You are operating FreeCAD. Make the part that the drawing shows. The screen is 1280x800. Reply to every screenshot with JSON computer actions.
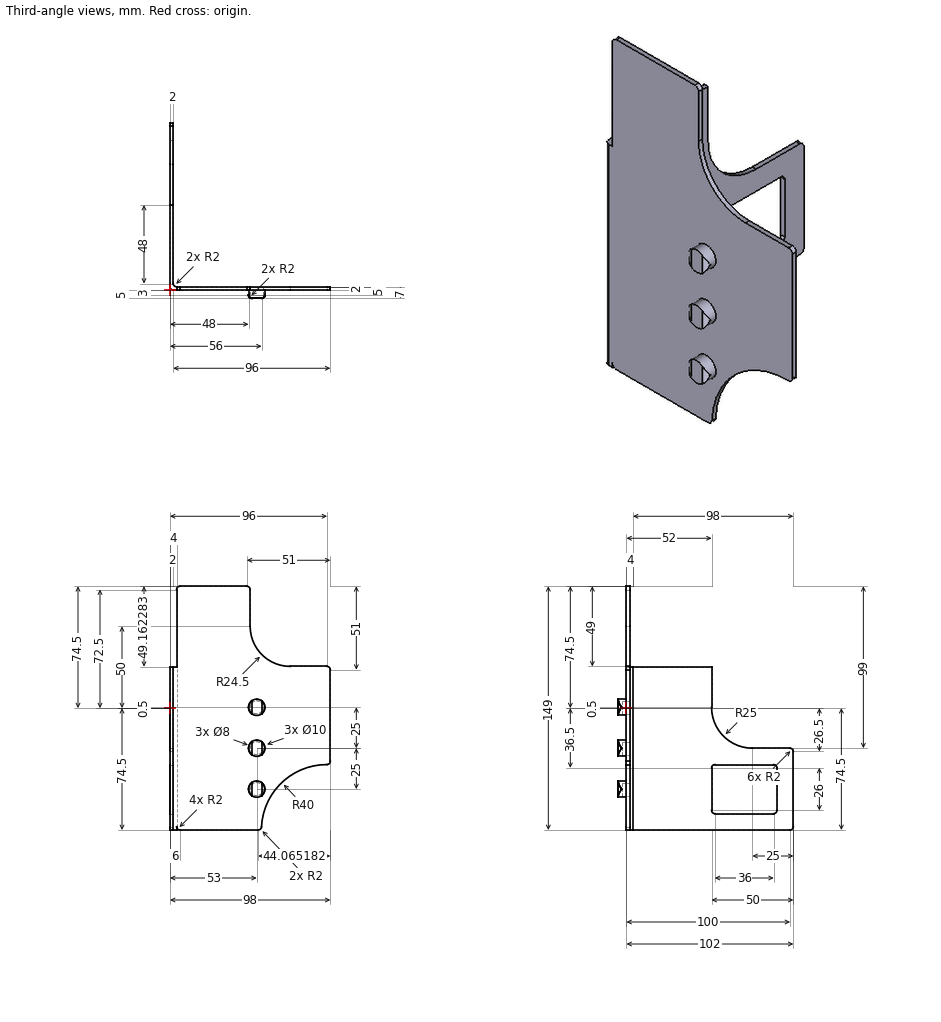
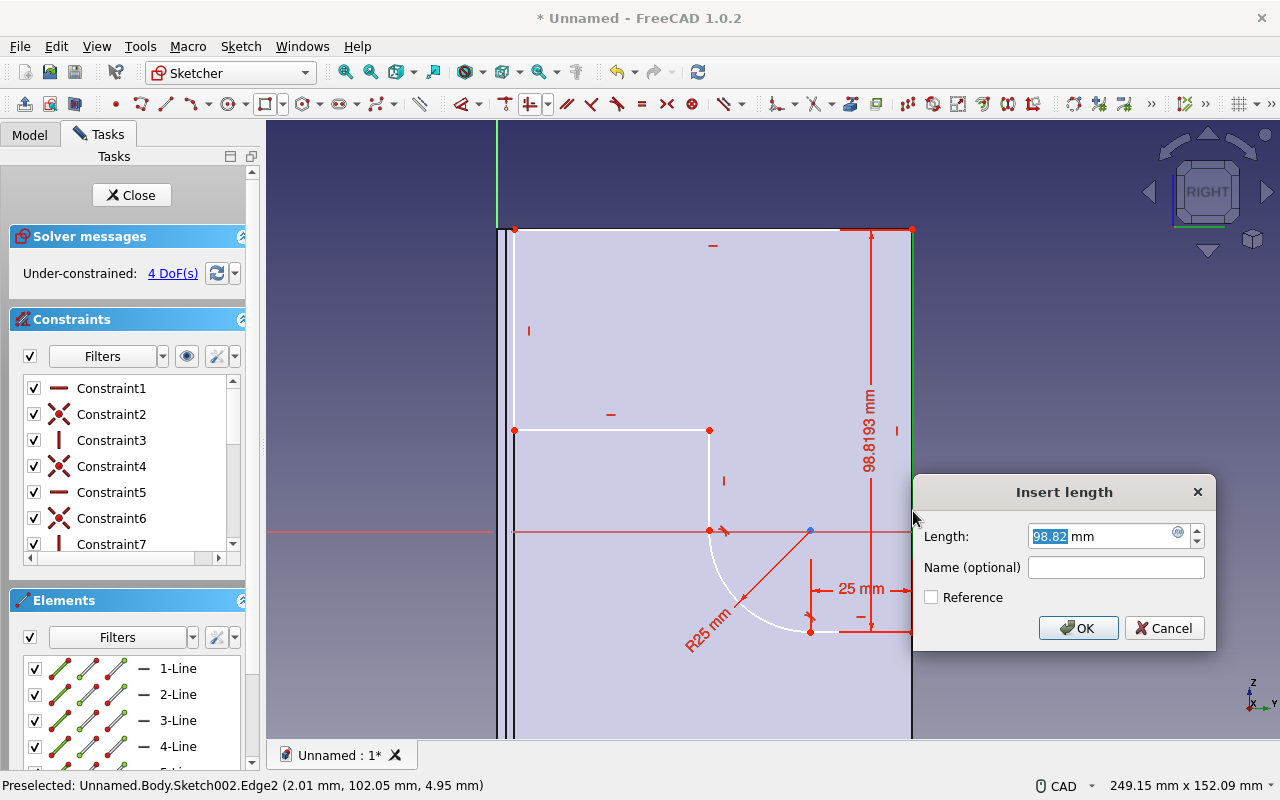
{"action": "type", "text": "99"}
{"action": "key", "text": "Return"}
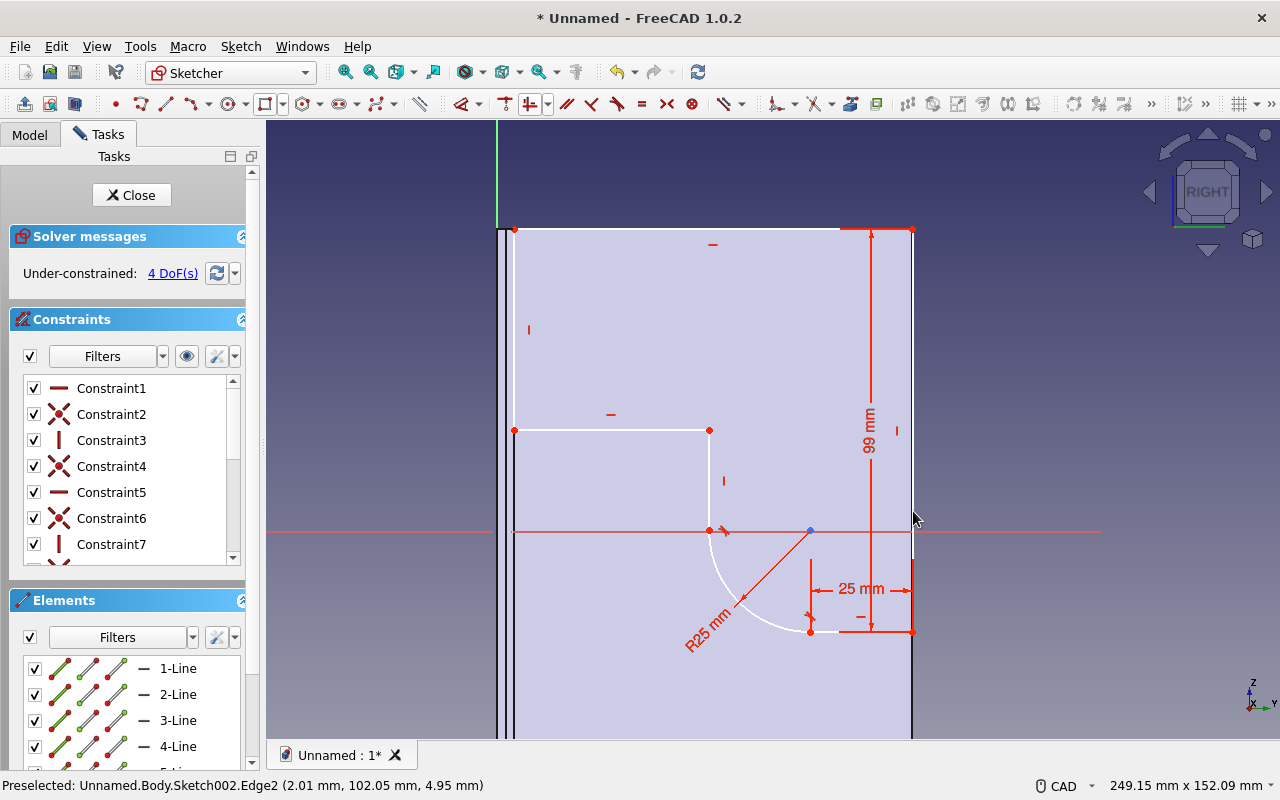
{"action": "left_click", "coordinate": [793, 229]}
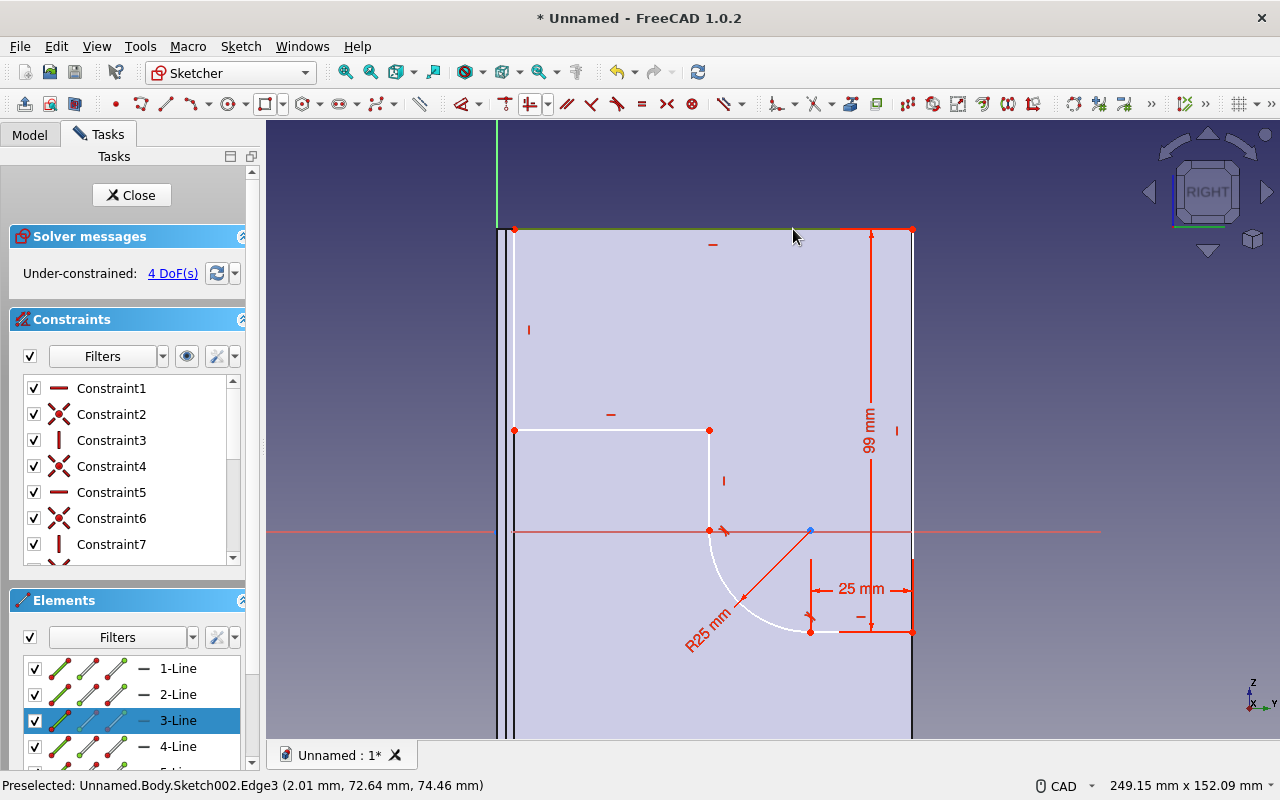
{"action": "left_click", "coordinate": [478, 104]}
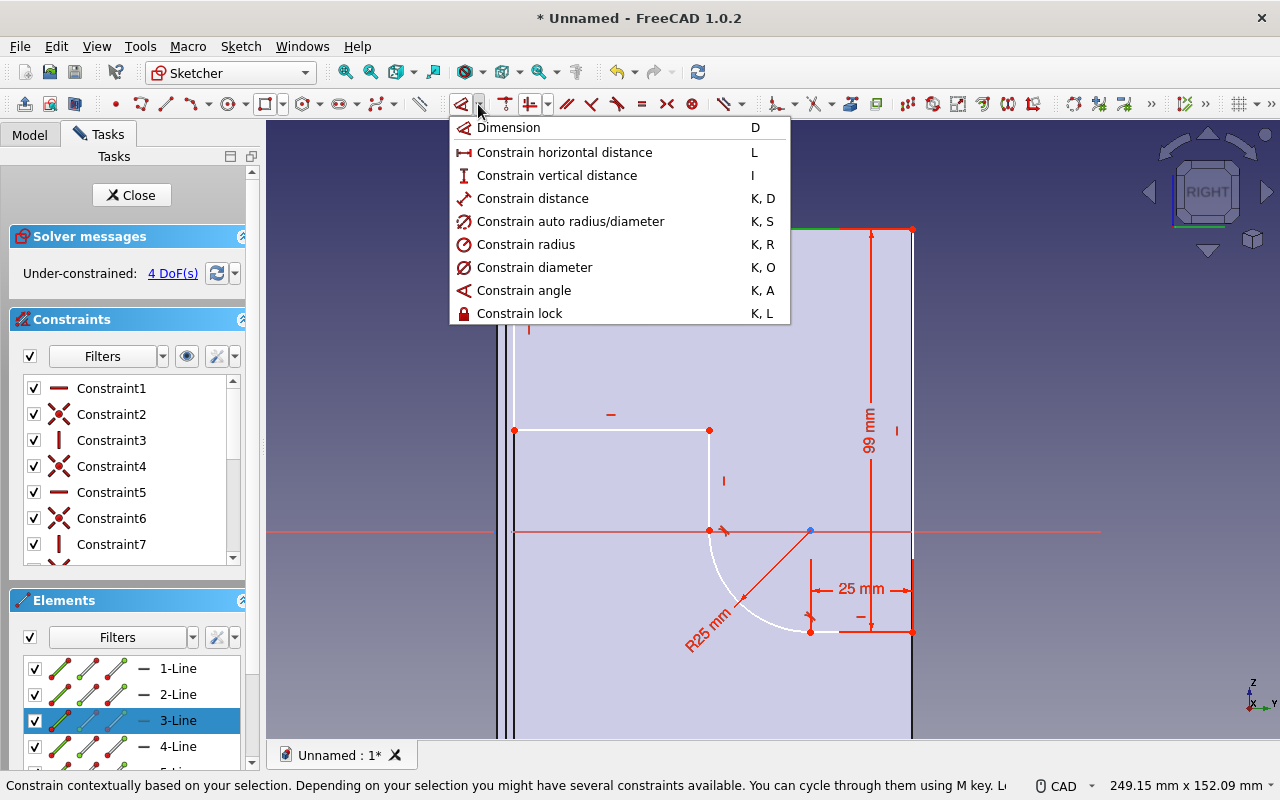
{"action": "left_click", "coordinate": [620, 152]}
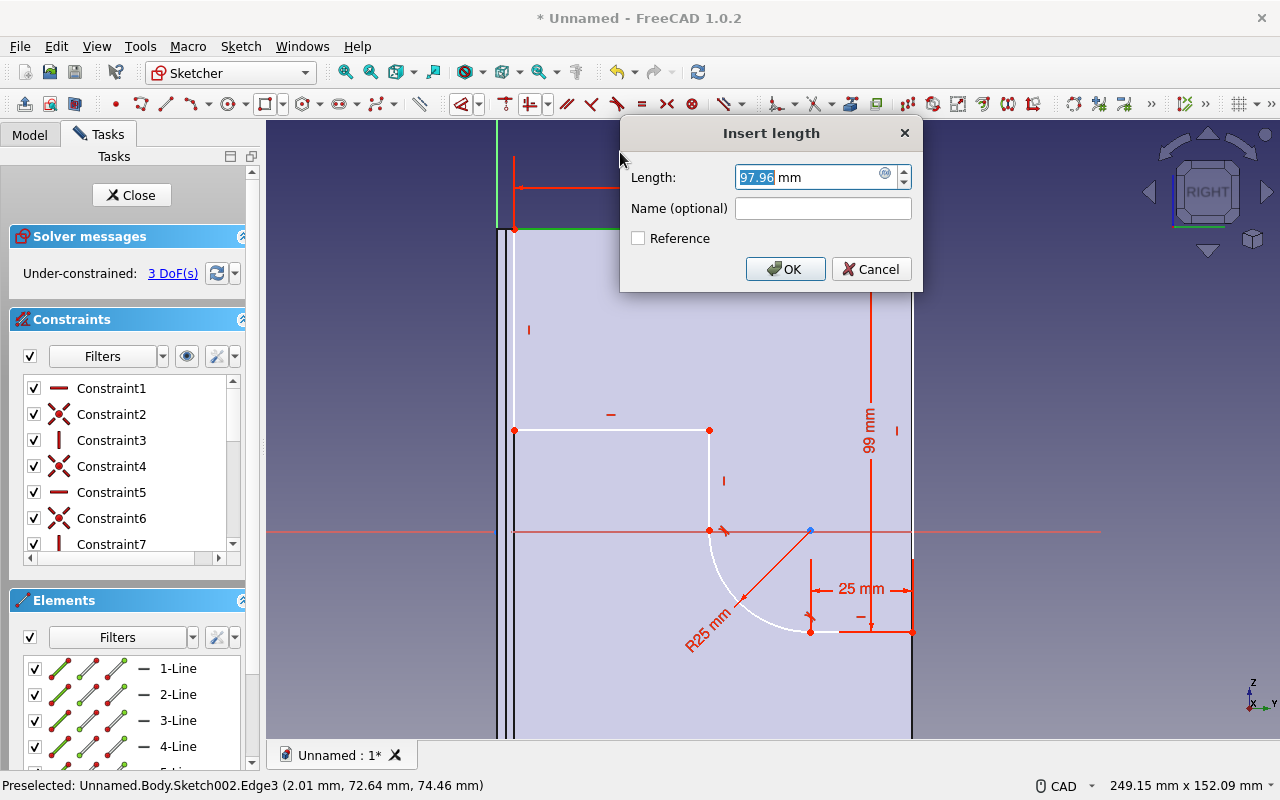
{"action": "type", "text": "98"}
{"action": "key", "text": "Return"}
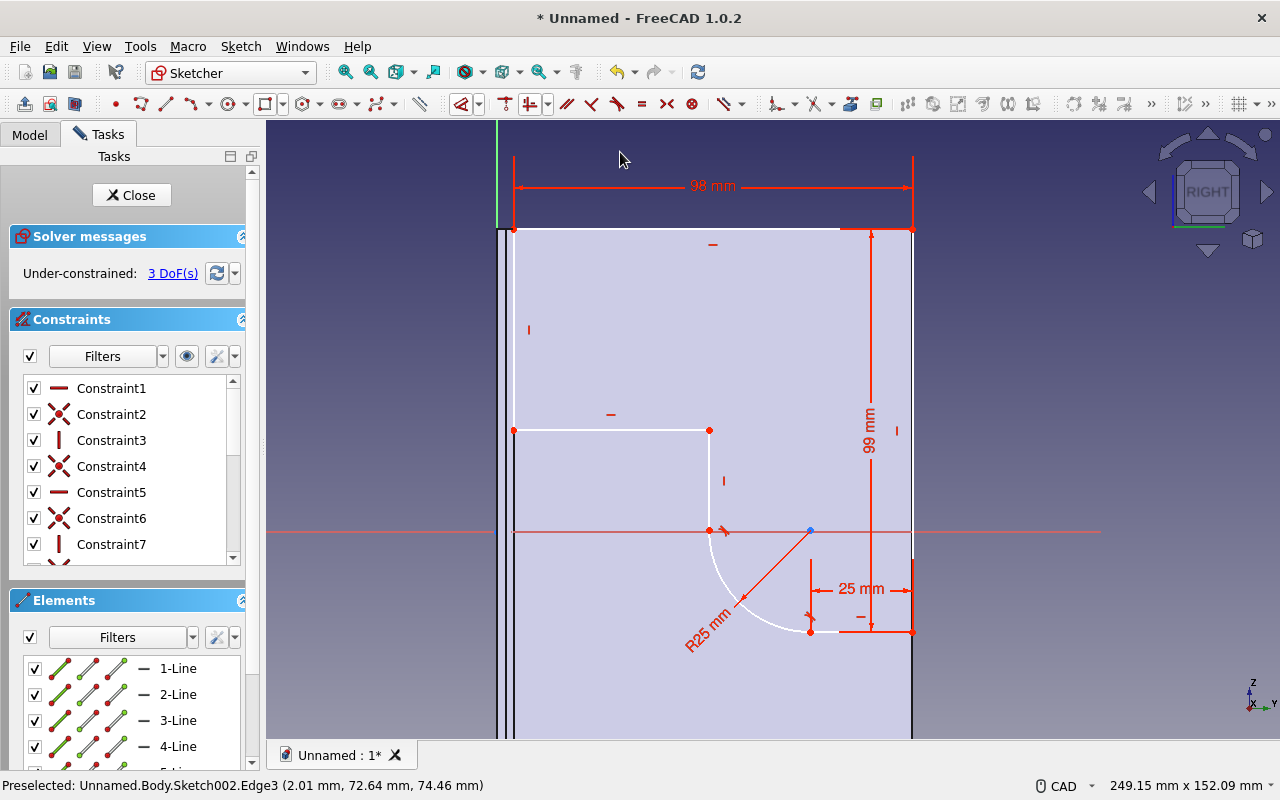
{"action": "left_click", "coordinate": [514, 289]}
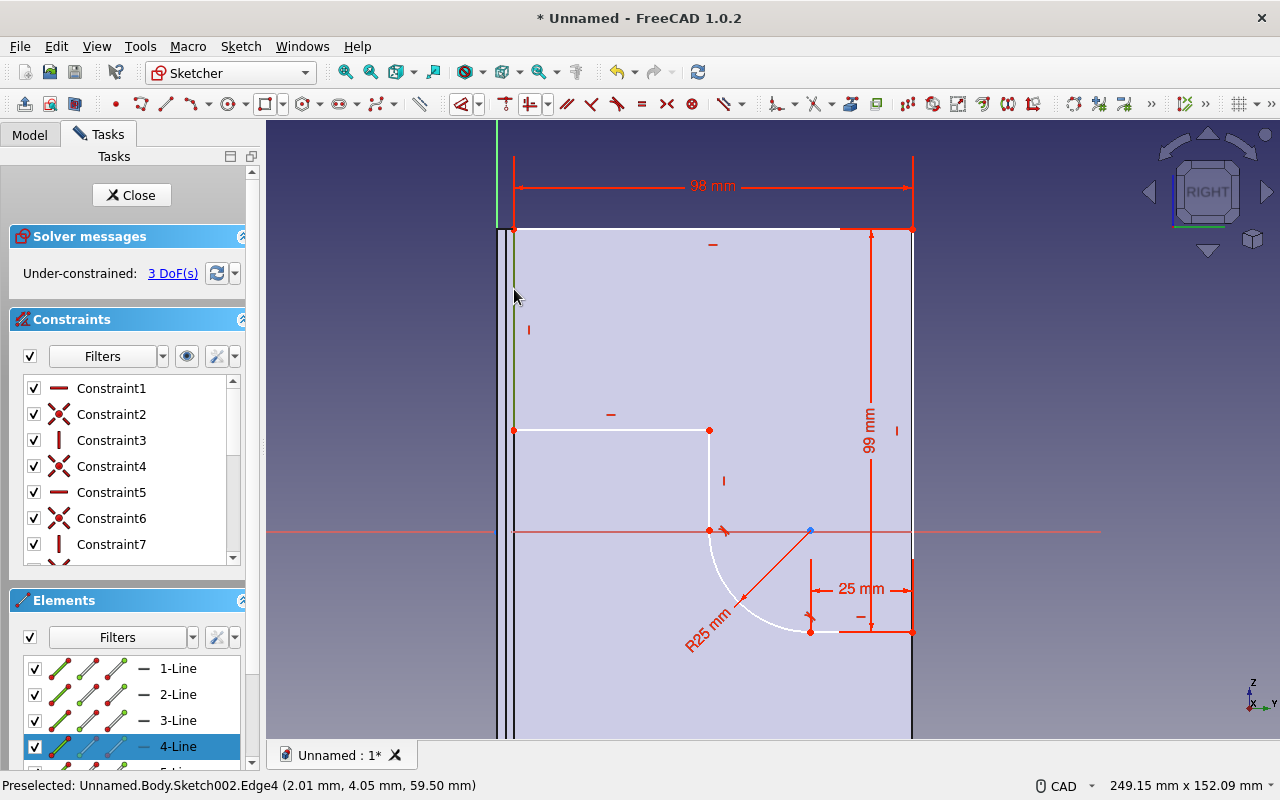
{"action": "key", "text": "i"}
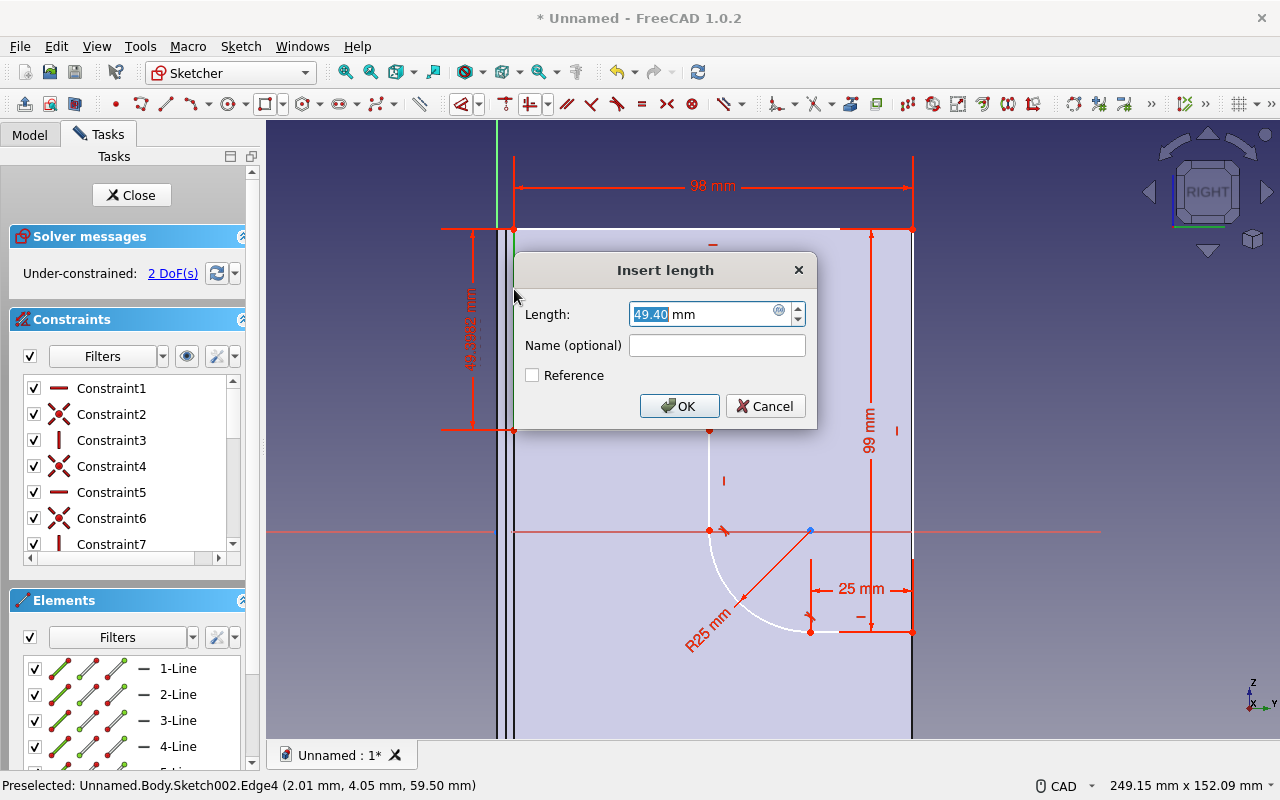
{"action": "type", "text": "49"}
{"action": "key", "text": "Return"}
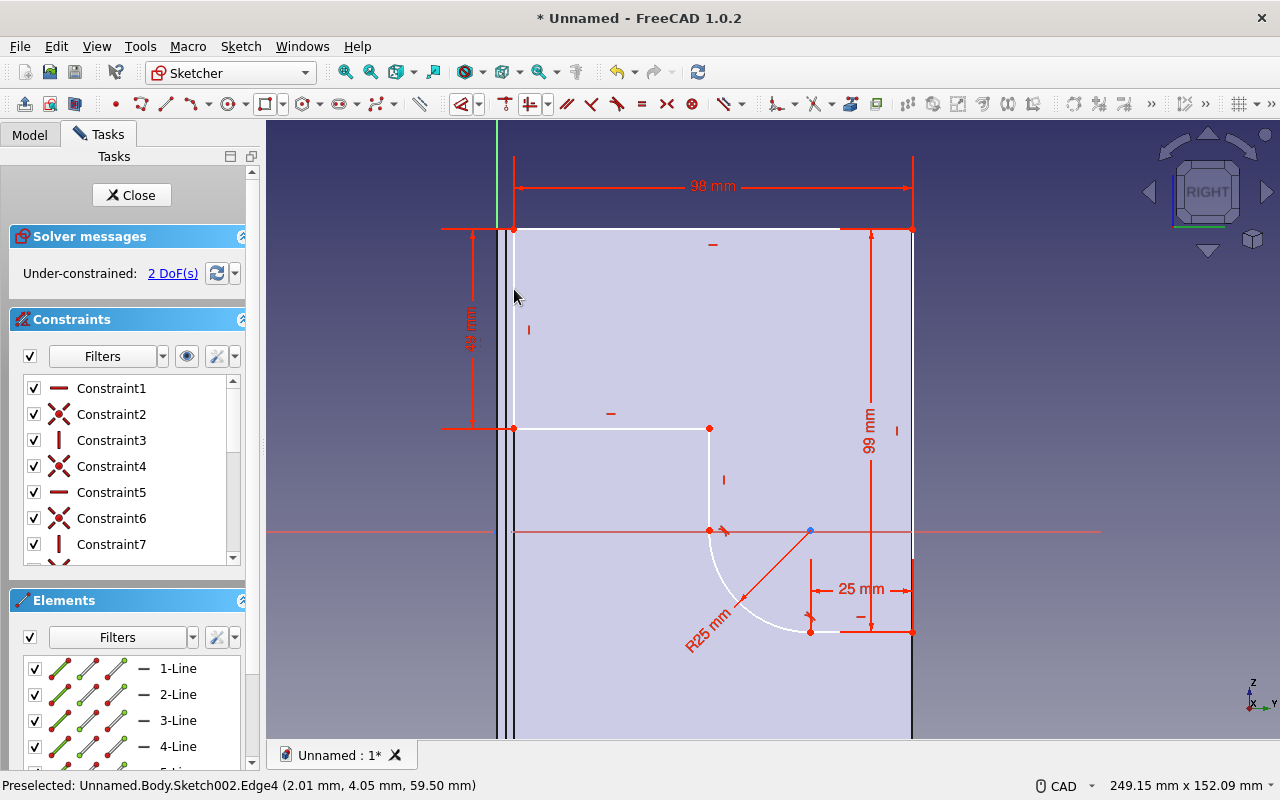
{"action": "scroll", "coordinate": [514, 229], "scroll_direction": "up", "scroll_amount": 5}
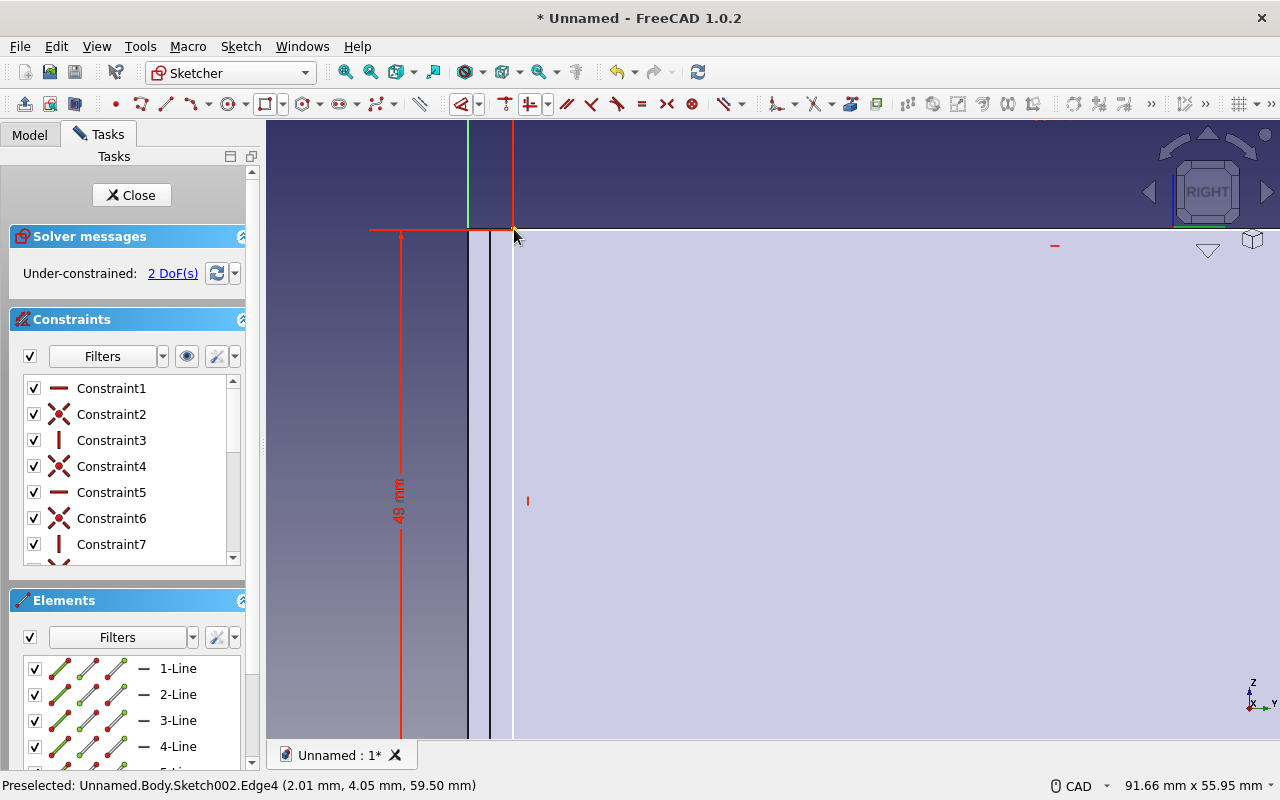
{"action": "left_click", "coordinate": [513, 230]}